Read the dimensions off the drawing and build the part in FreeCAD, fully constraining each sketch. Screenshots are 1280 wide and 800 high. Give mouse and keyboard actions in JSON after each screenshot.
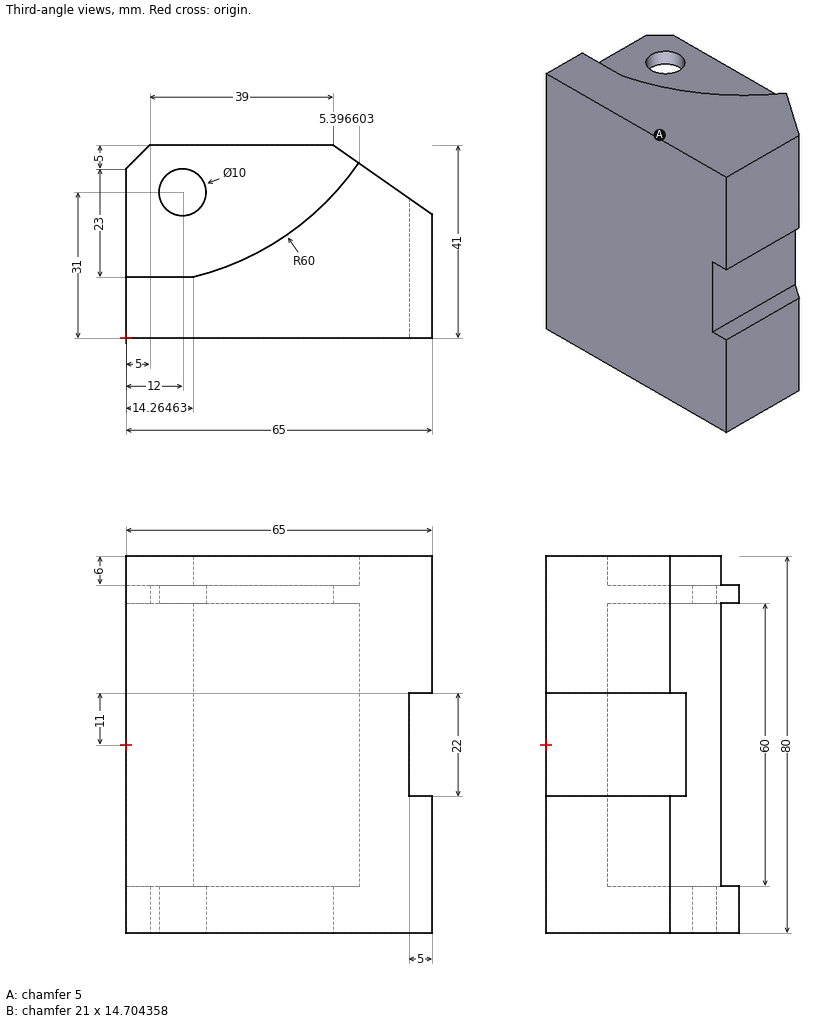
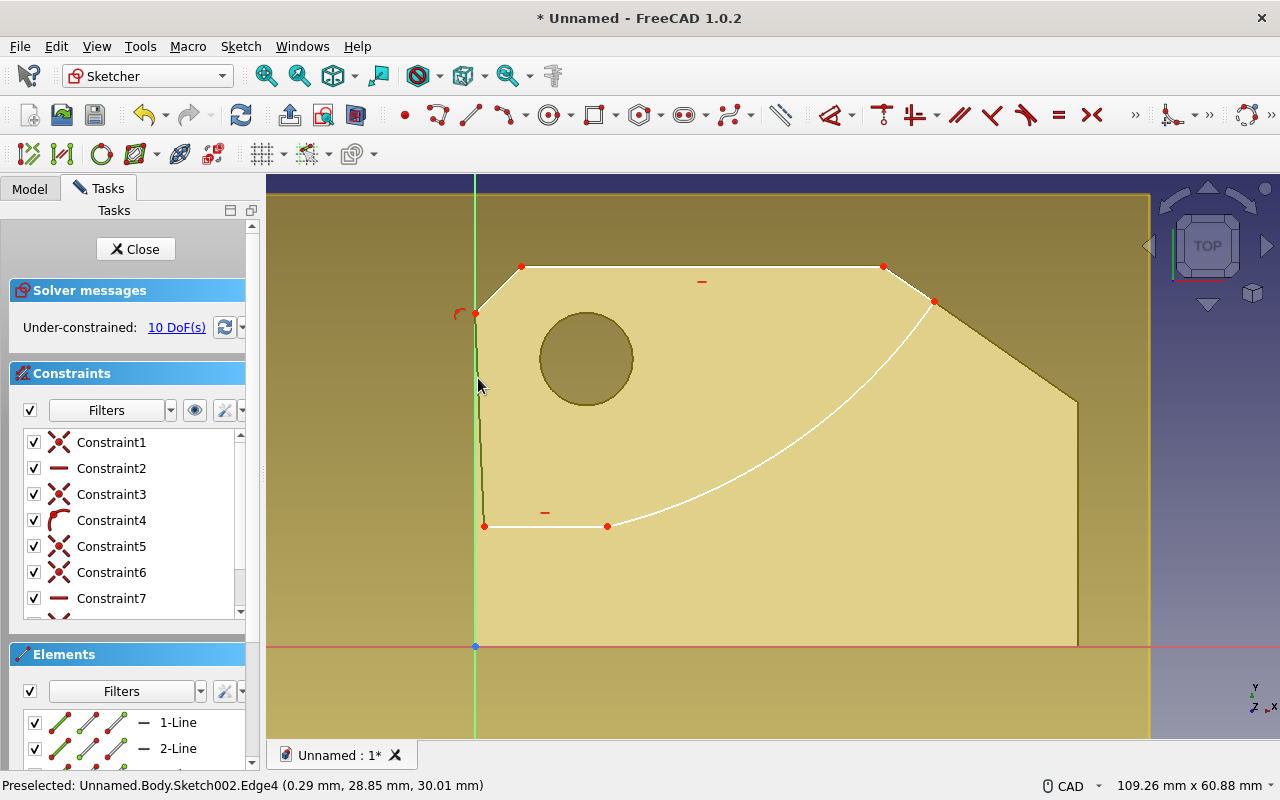
{"action": "key", "text": "v"}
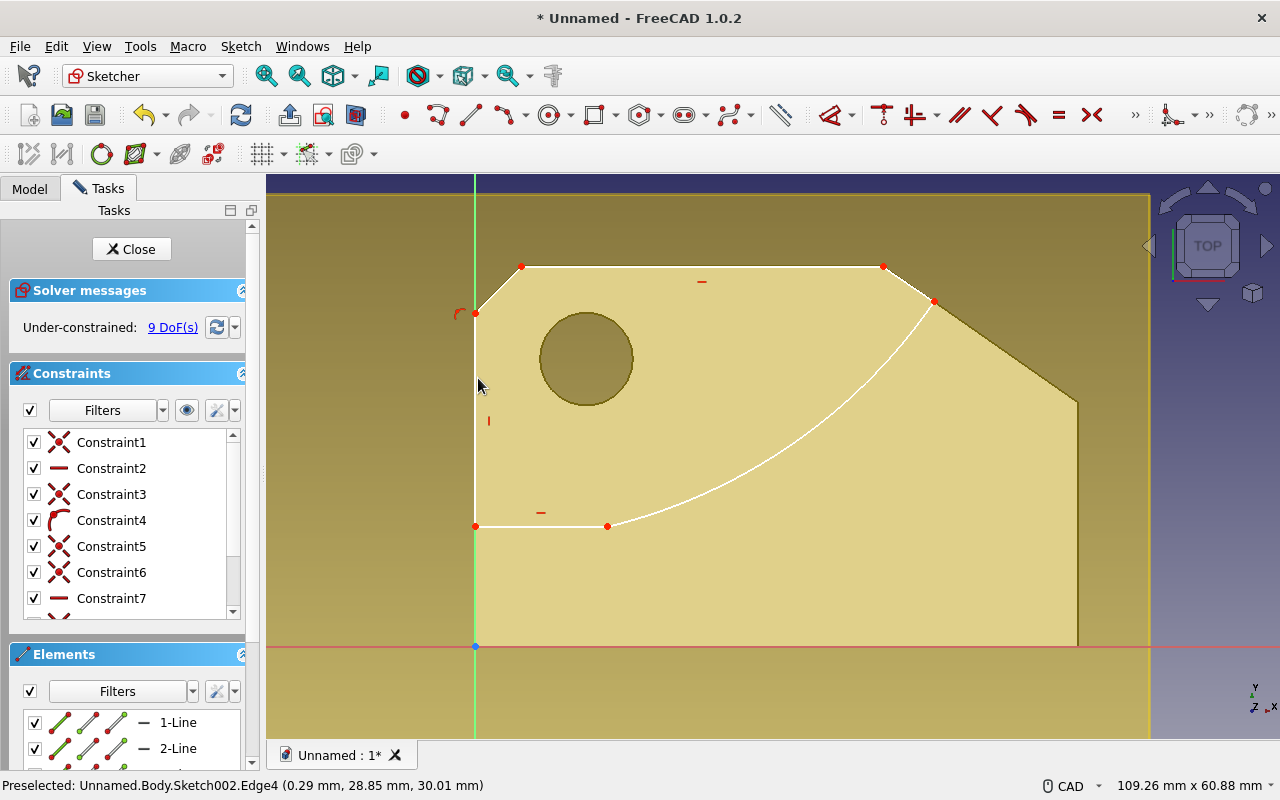
{"action": "scroll", "coordinate": [705, 626], "scroll_direction": "down", "scroll_amount": 3}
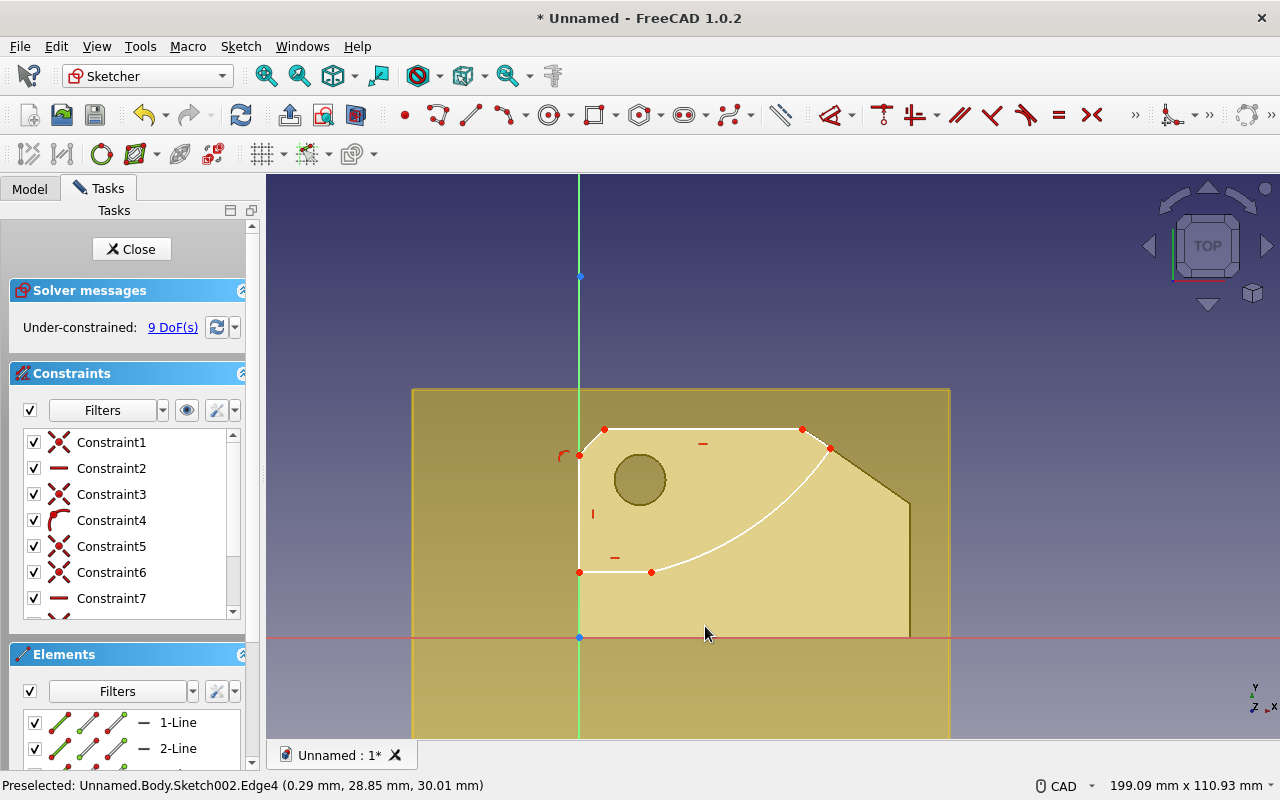
{"action": "left_click", "coordinate": [580, 276]}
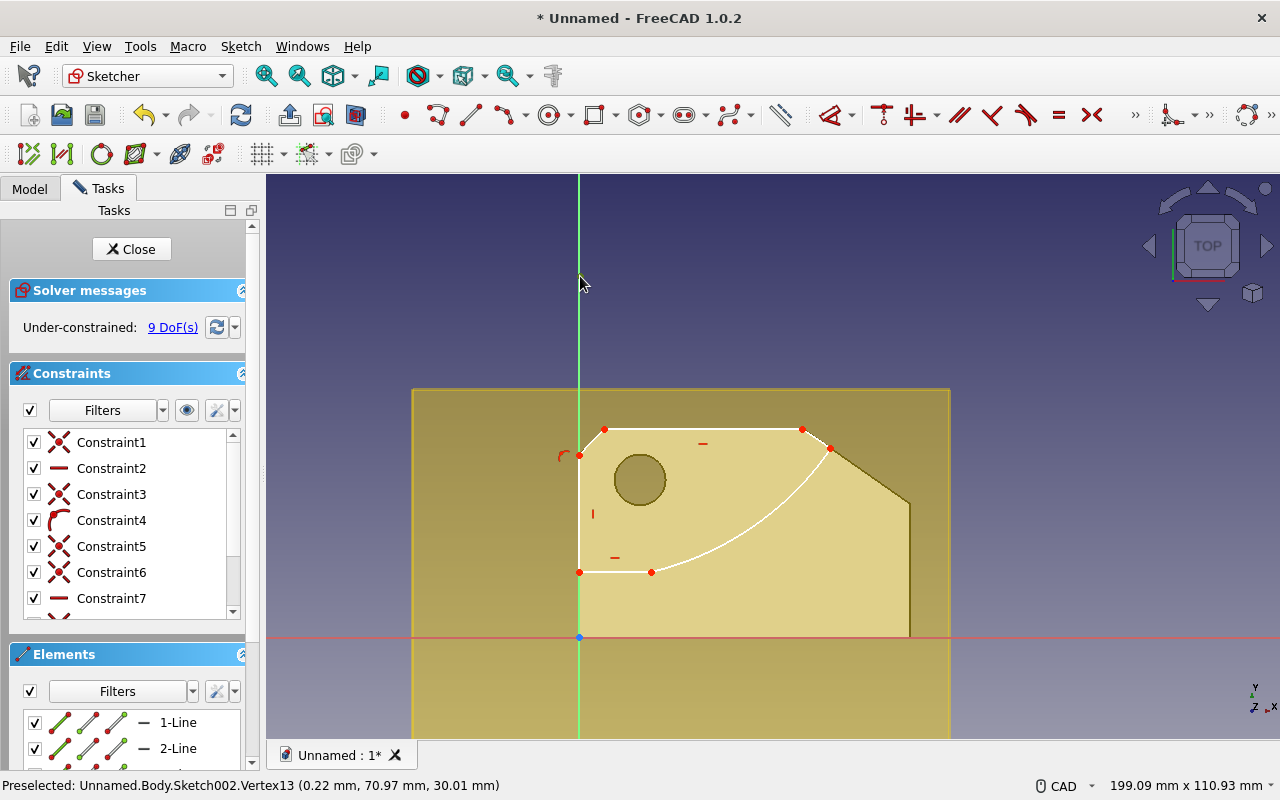
{"action": "left_click", "coordinate": [579, 675]}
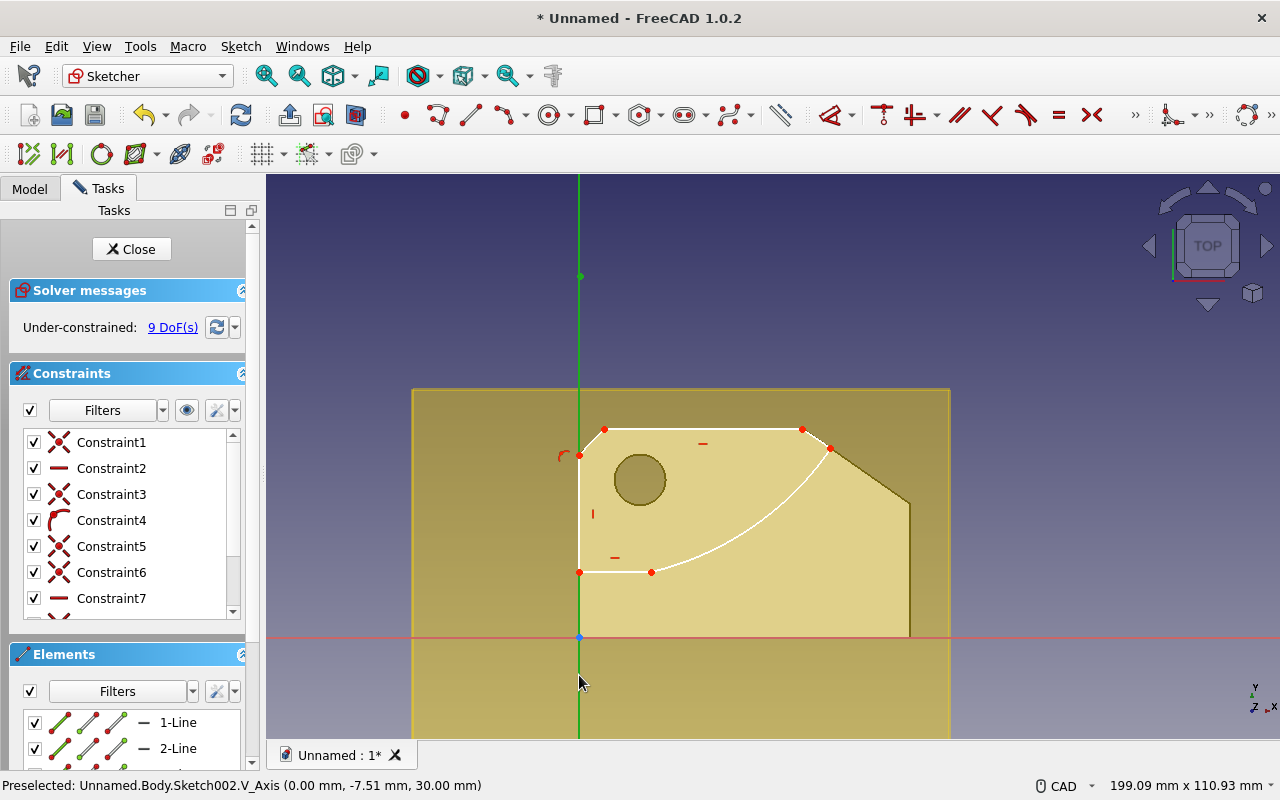
{"action": "key", "text": "c"}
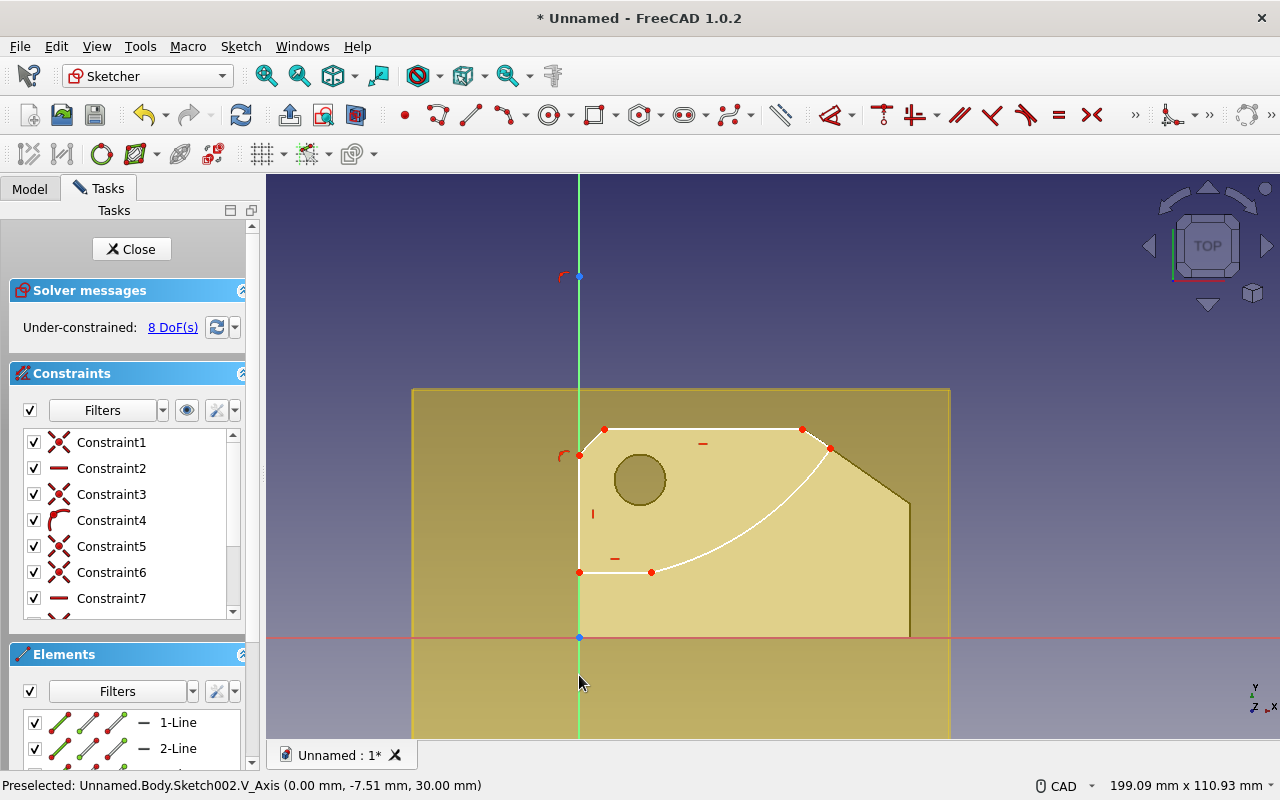
{"action": "key", "text": "d"}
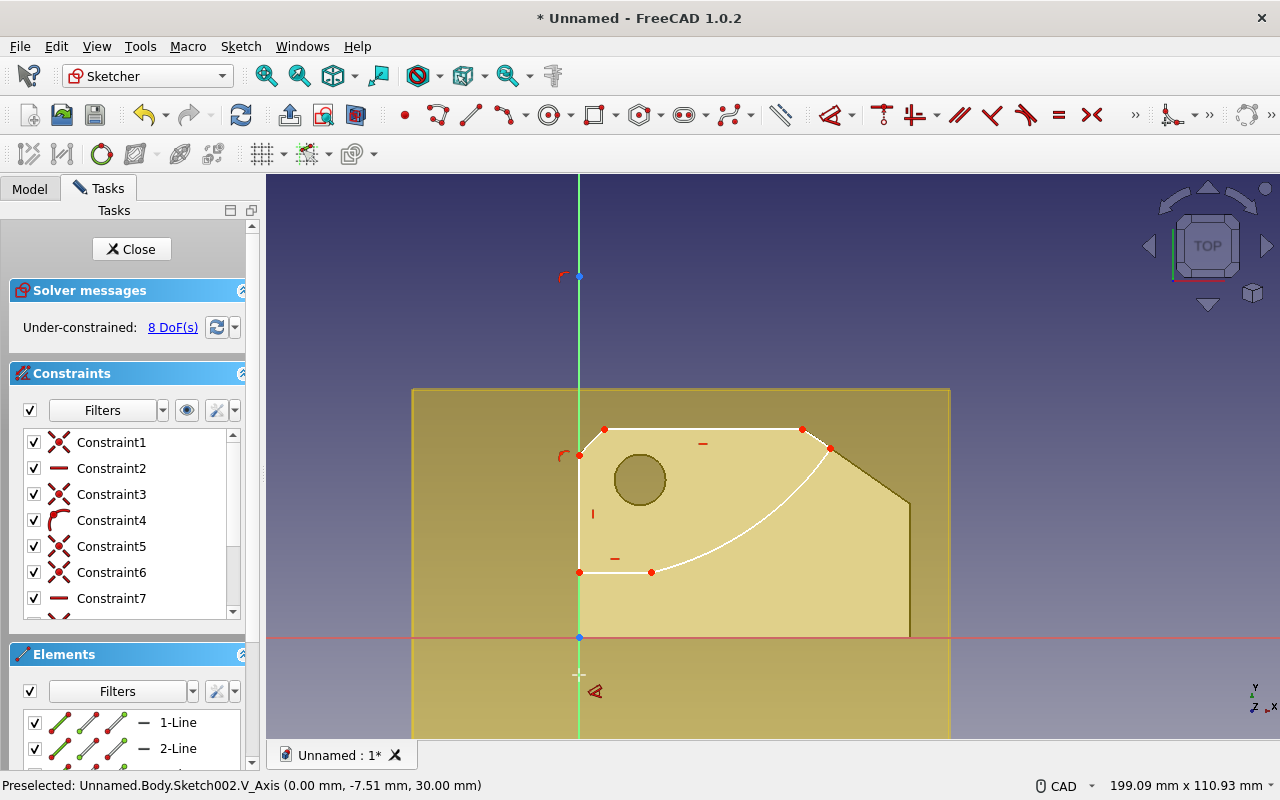
{"action": "left_click", "coordinate": [714, 550]}
{"action": "left_click", "coordinate": [728, 579]}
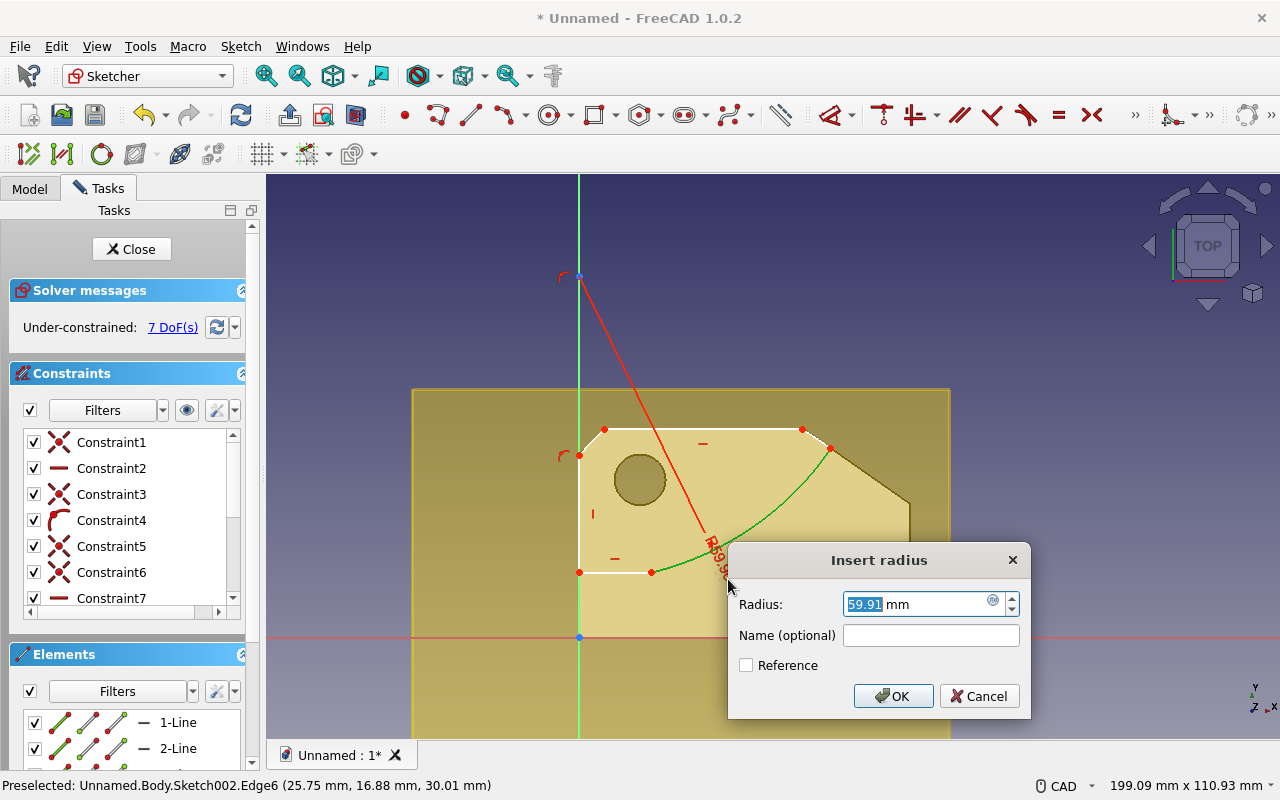
{"action": "type", "text": "60"}
{"action": "key", "text": "Return"}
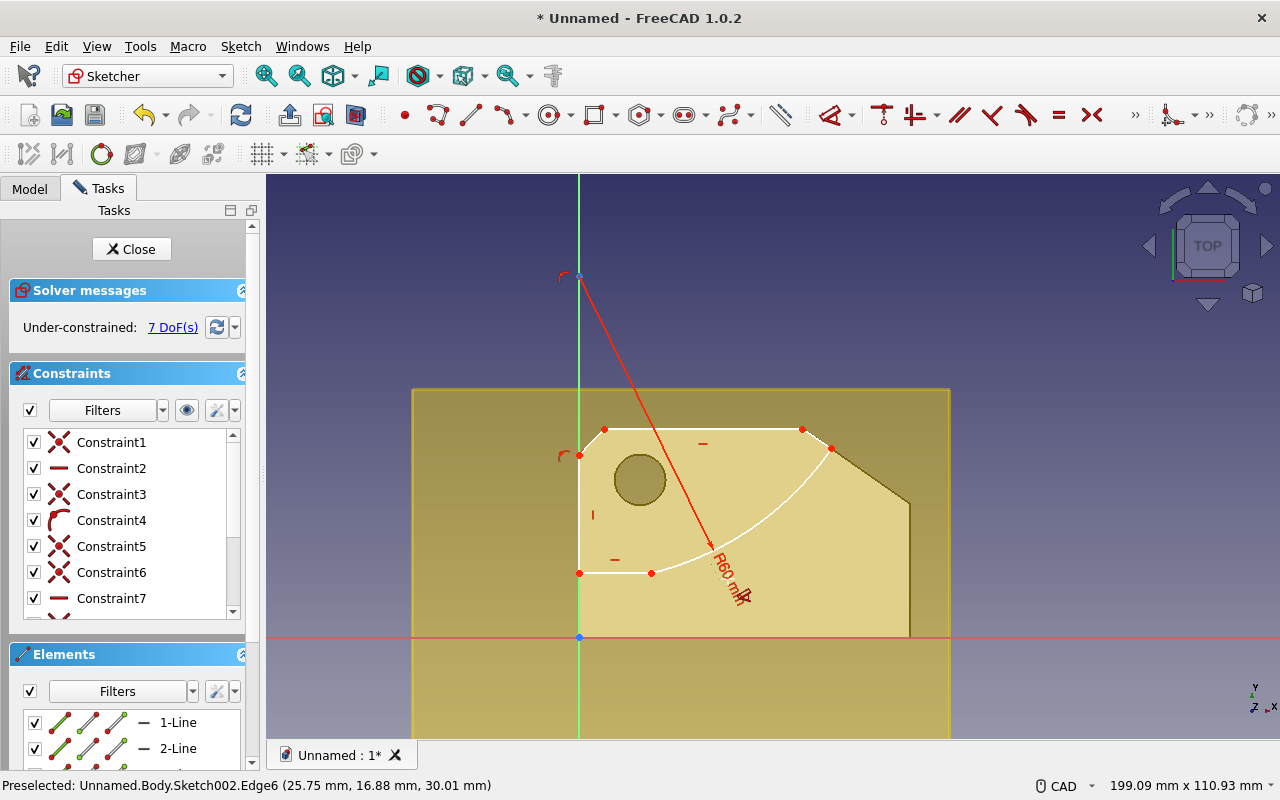
{"action": "left_click", "coordinate": [743, 429]}
{"action": "left_click", "coordinate": [704, 395]}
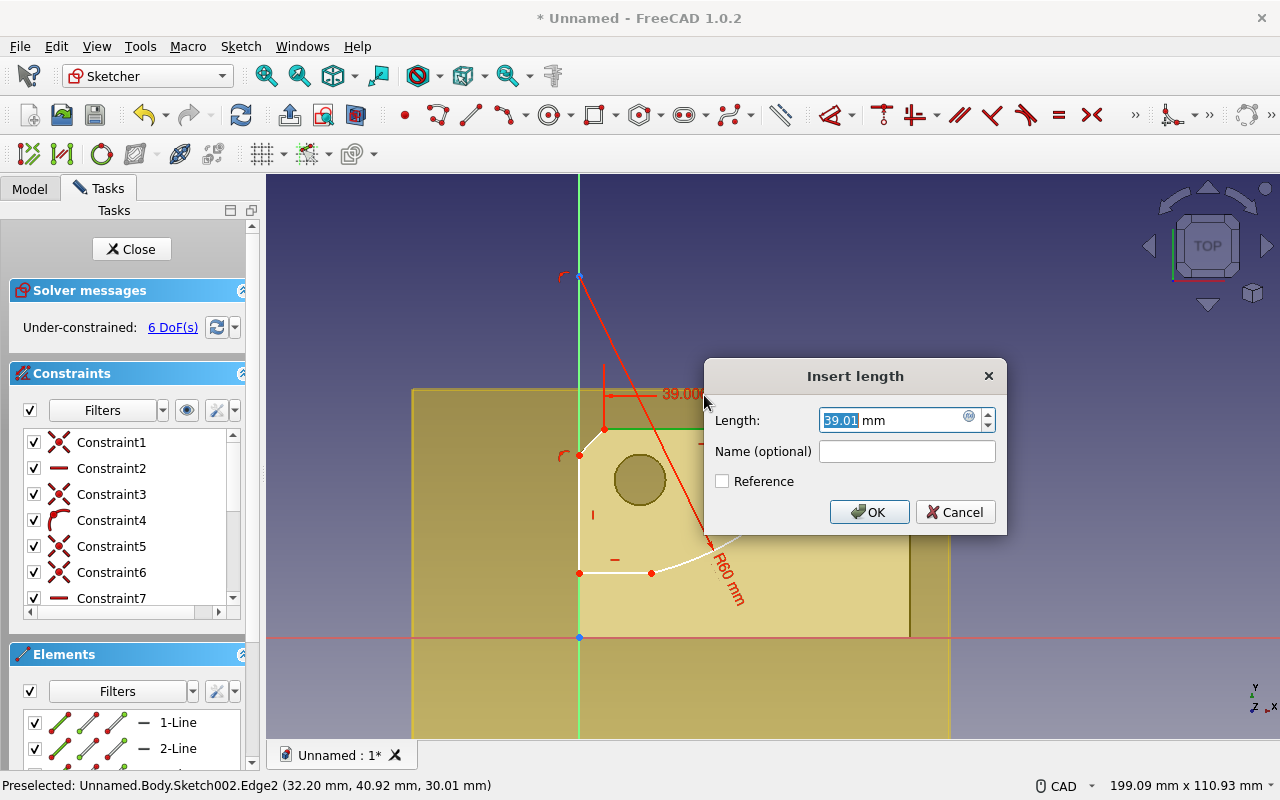
{"action": "type", "text": "39"}
{"action": "key", "text": "Return"}